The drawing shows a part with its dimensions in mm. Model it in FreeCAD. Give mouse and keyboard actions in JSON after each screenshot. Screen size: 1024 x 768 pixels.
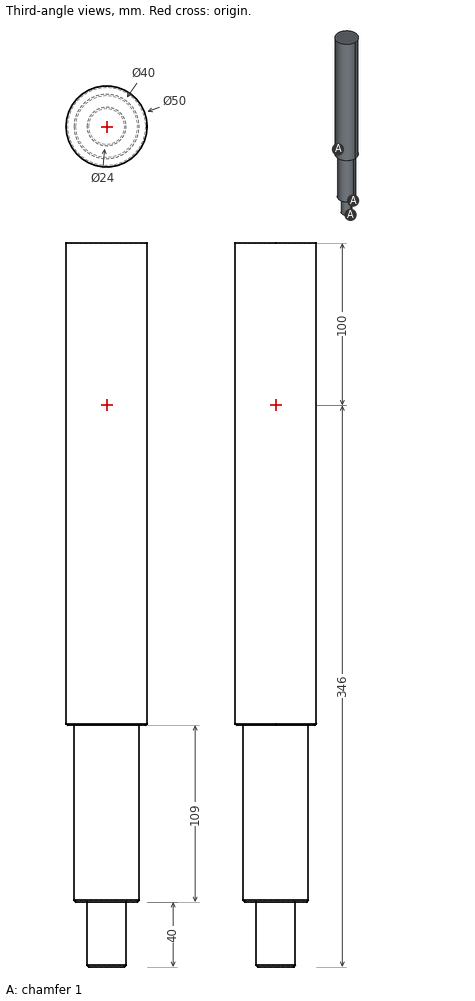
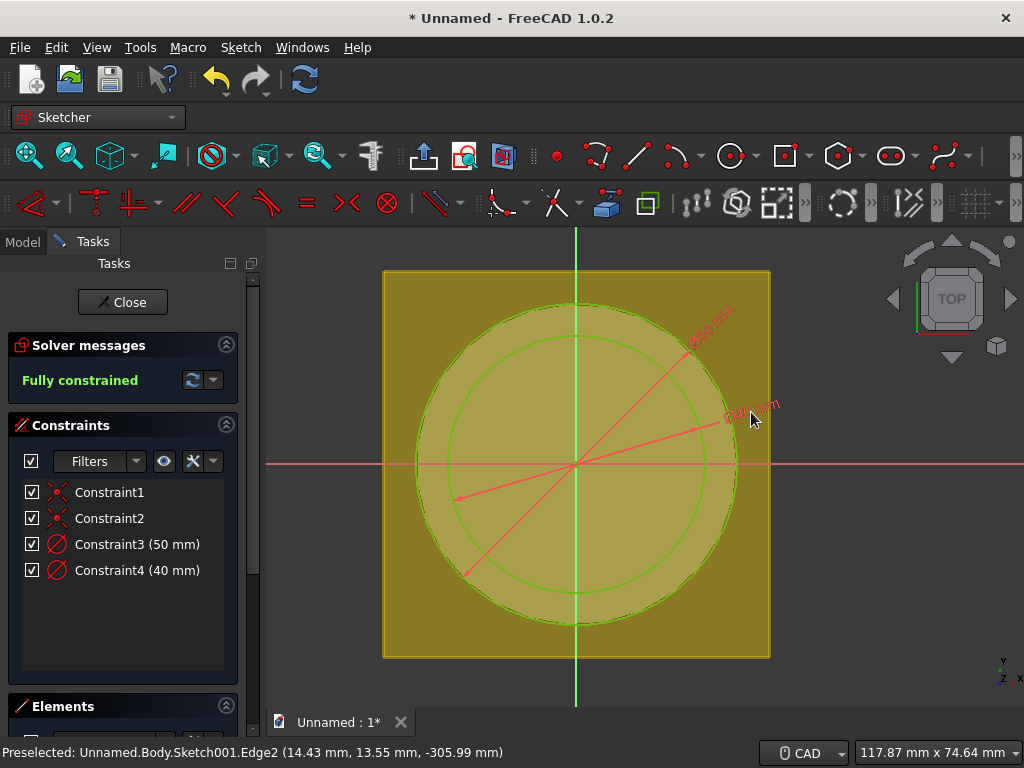
{"action": "left_click", "coordinate": [123, 302]}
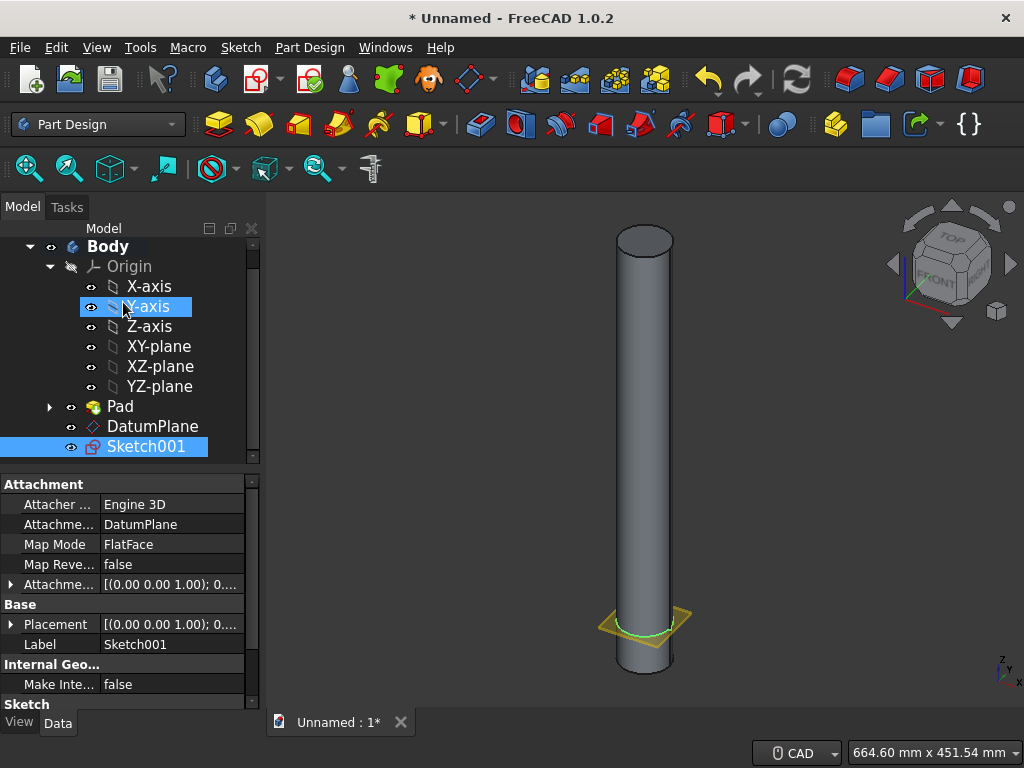
{"action": "left_click", "coordinate": [482, 124]}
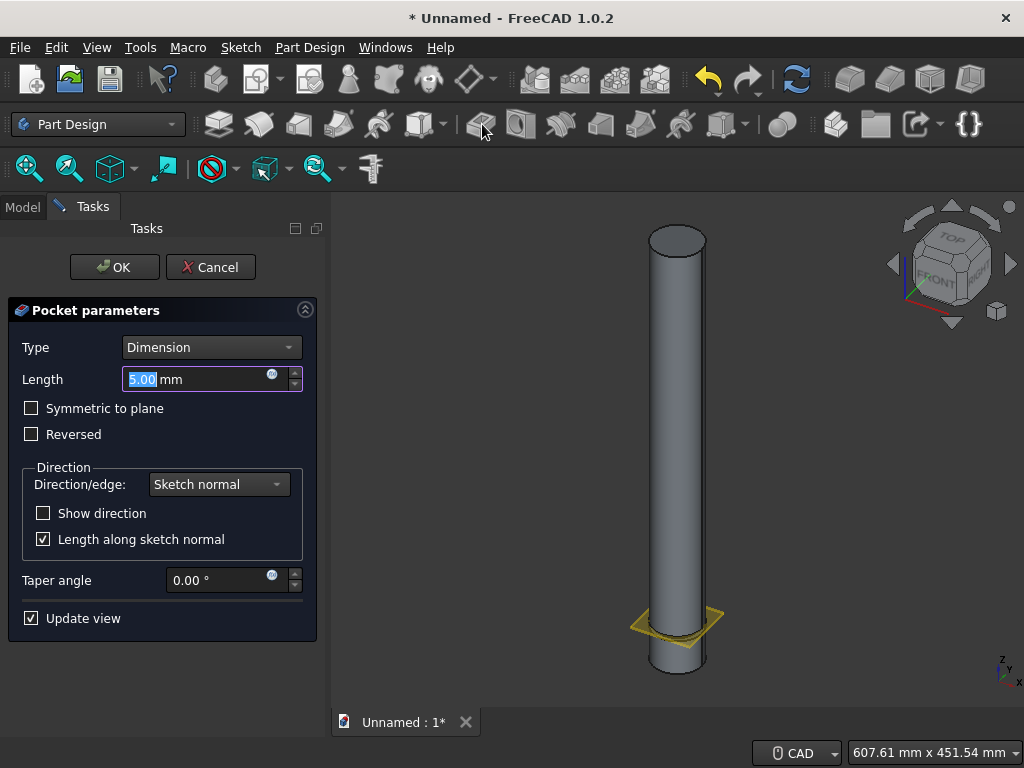
{"action": "type", "text": "109"}
{"action": "key", "text": "Tab"}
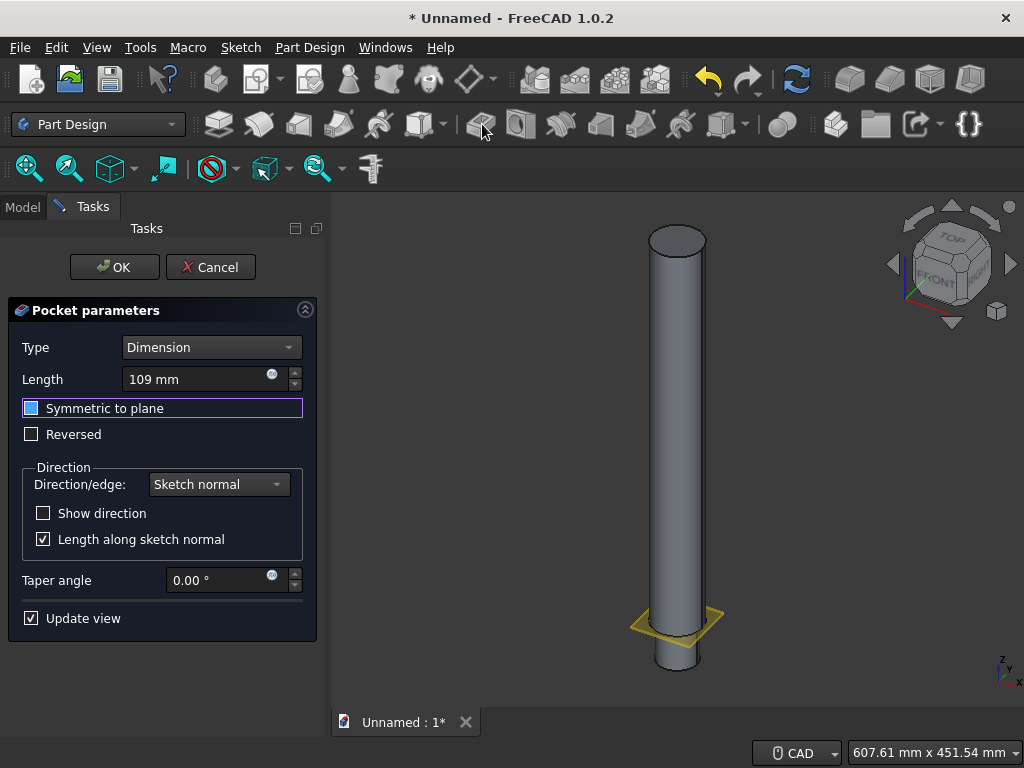
{"action": "left_click", "coordinate": [30, 434]}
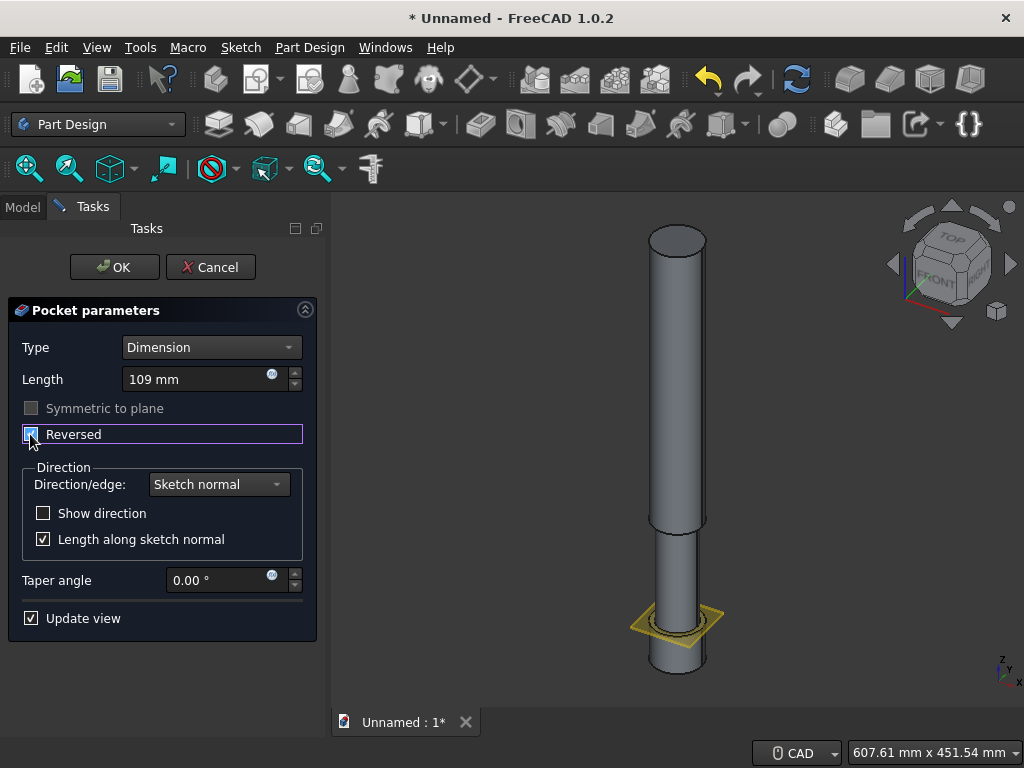
{"action": "left_click", "coordinate": [115, 267]}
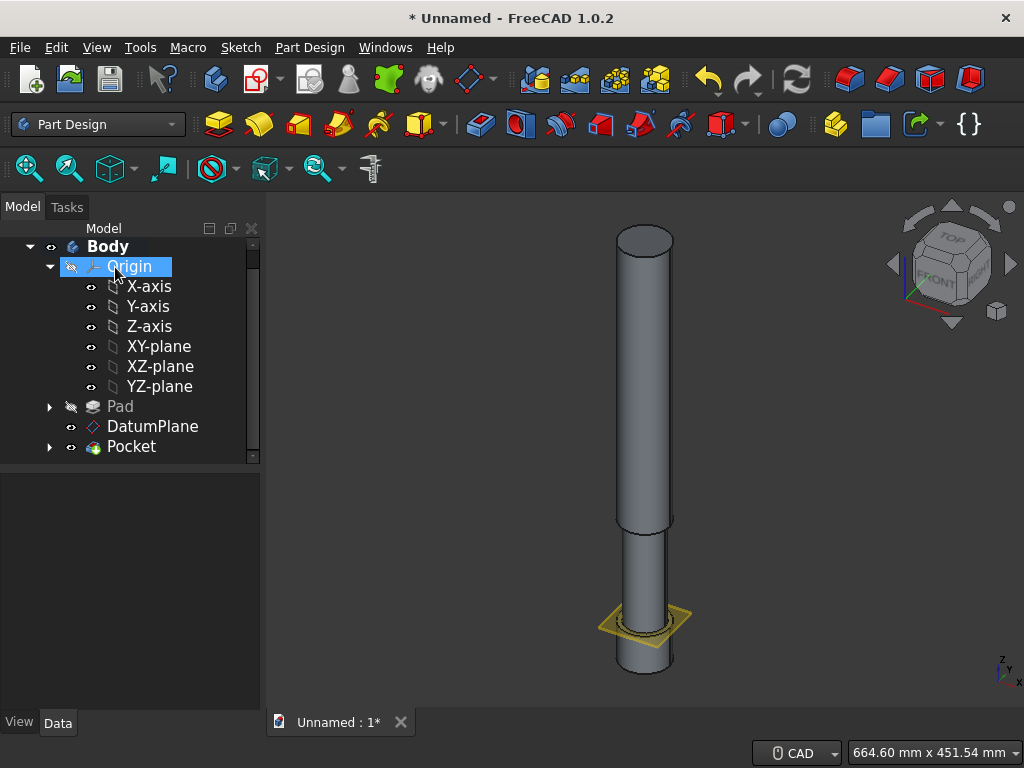
{"action": "left_click", "coordinate": [116, 427]}
{"action": "key", "text": "space"}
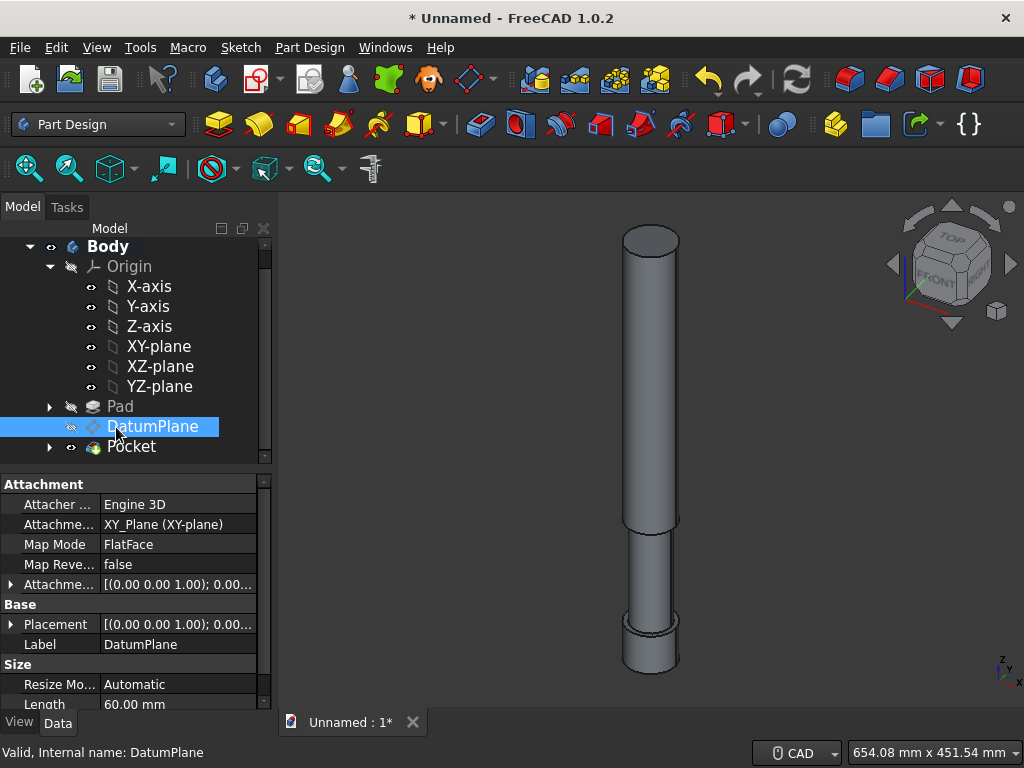
{"action": "key", "text": "5"}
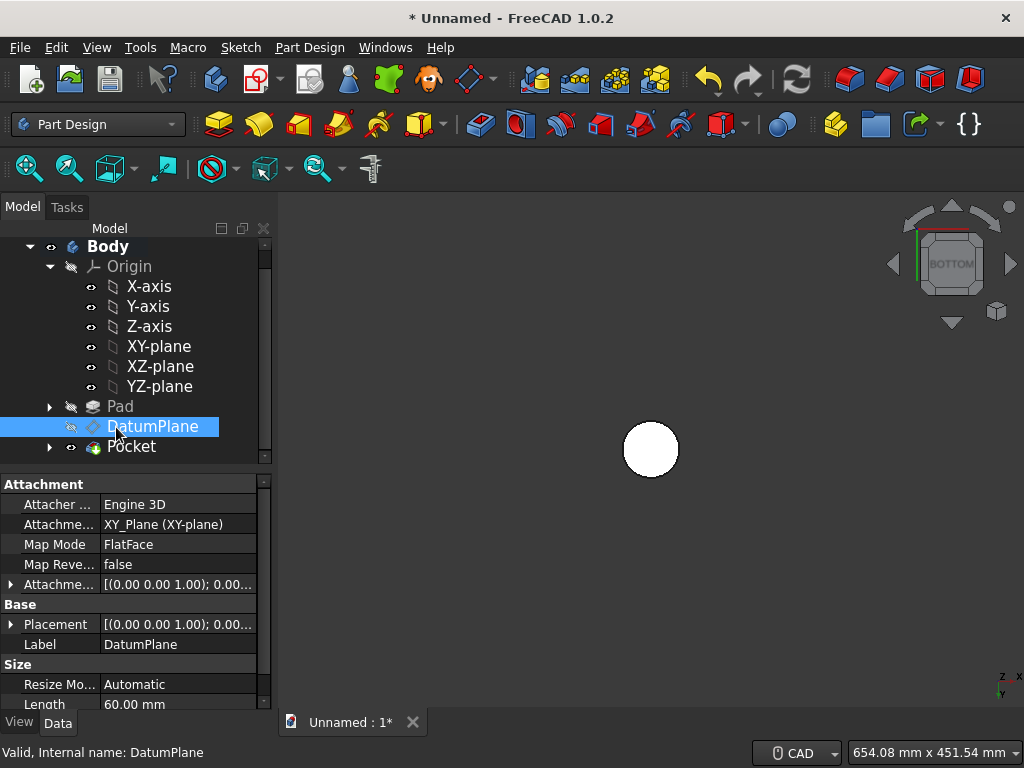
{"action": "left_click", "coordinate": [30, 170]}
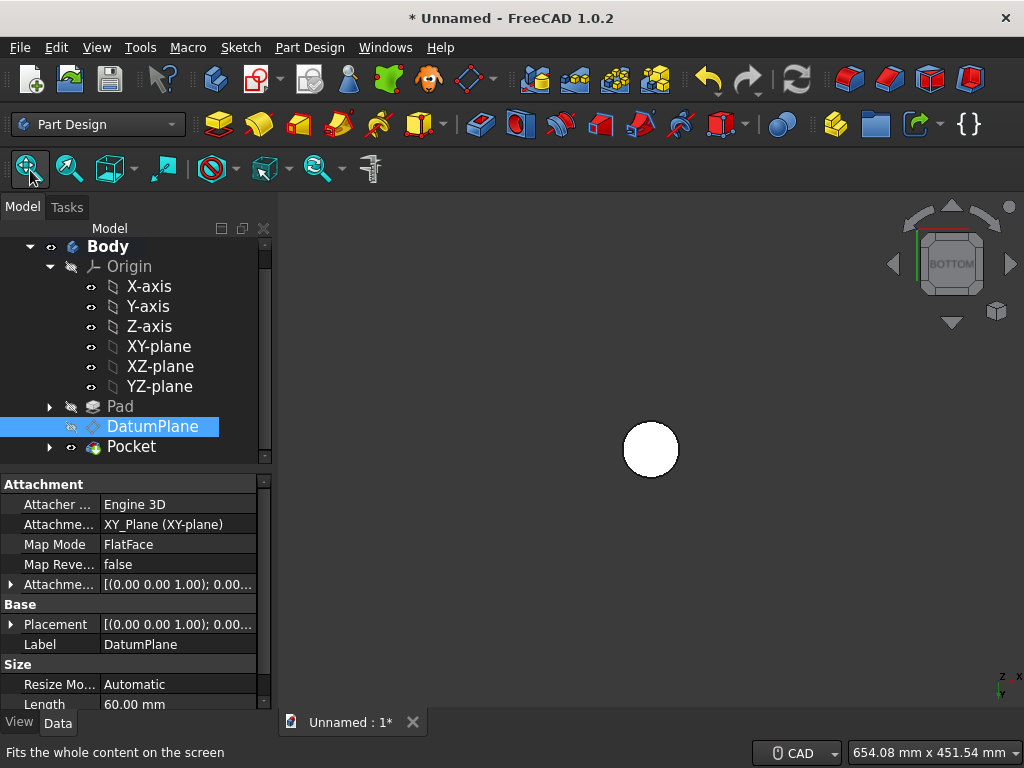
{"action": "left_click", "coordinate": [651, 448]}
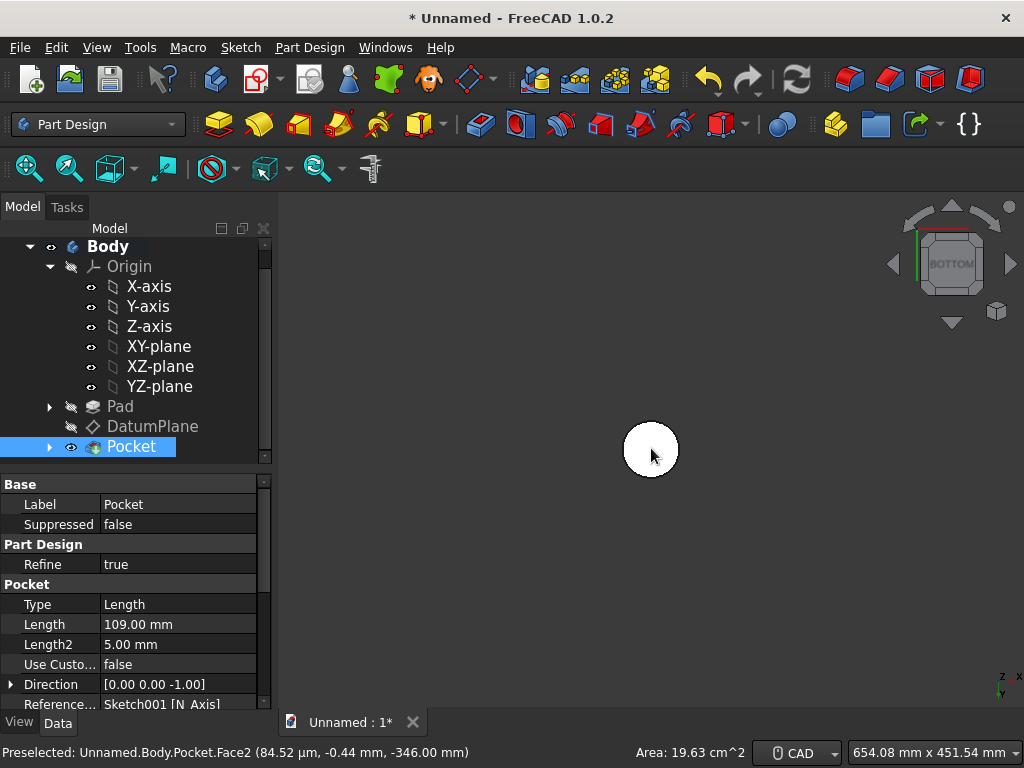
{"action": "left_click", "coordinate": [256, 80]}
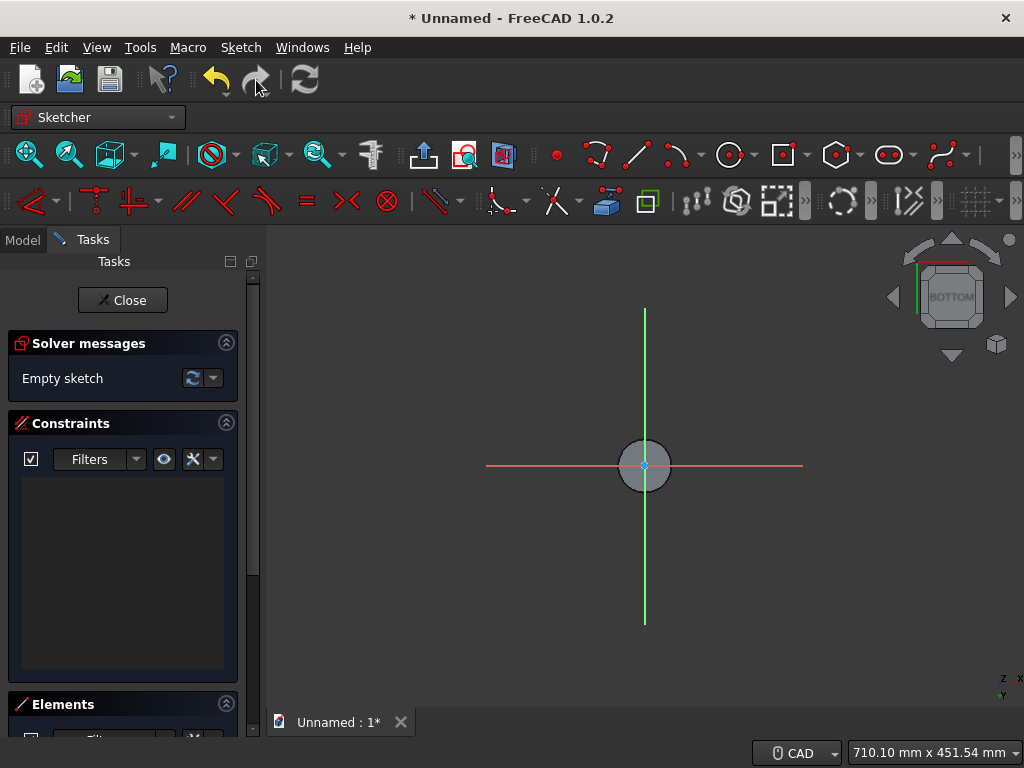
{"action": "scroll", "coordinate": [658, 466], "scroll_direction": "up", "scroll_amount": 9}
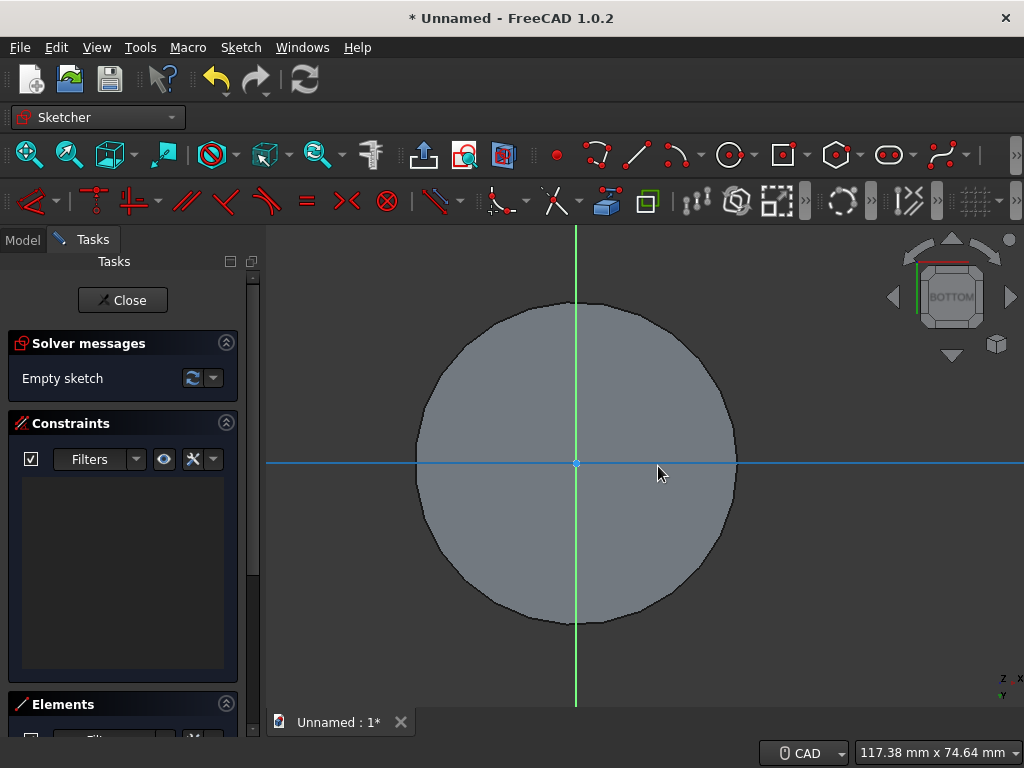
{"action": "left_click", "coordinate": [730, 156]}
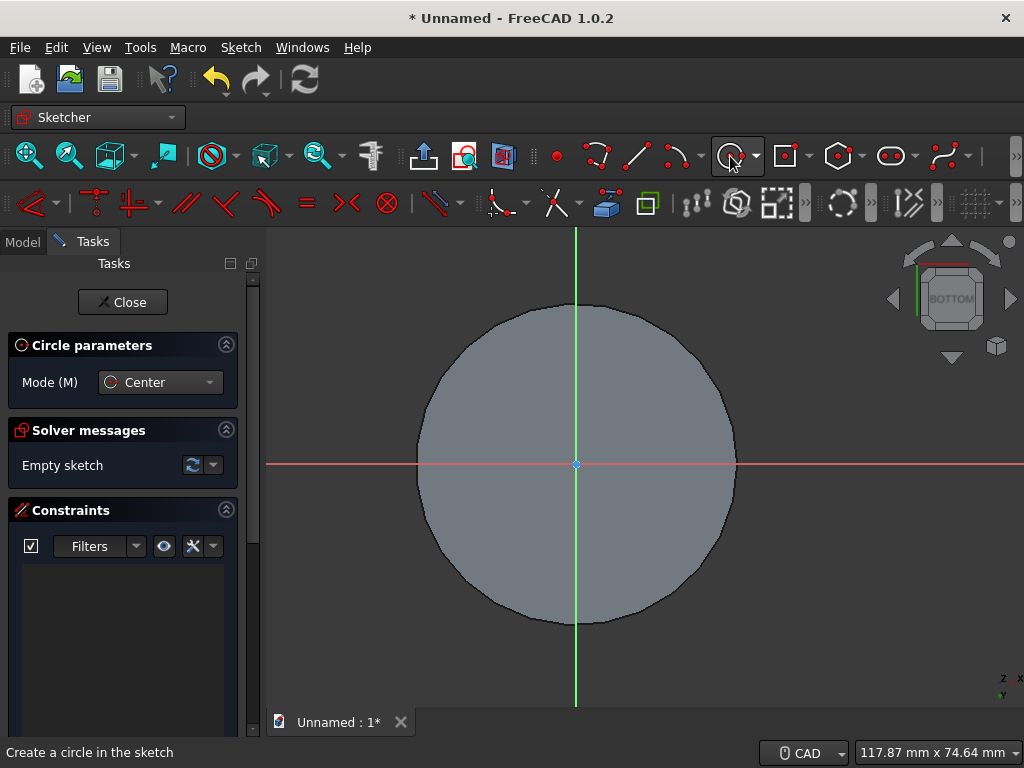
{"action": "left_click", "coordinate": [576, 464]}
{"action": "left_click", "coordinate": [690, 351]}